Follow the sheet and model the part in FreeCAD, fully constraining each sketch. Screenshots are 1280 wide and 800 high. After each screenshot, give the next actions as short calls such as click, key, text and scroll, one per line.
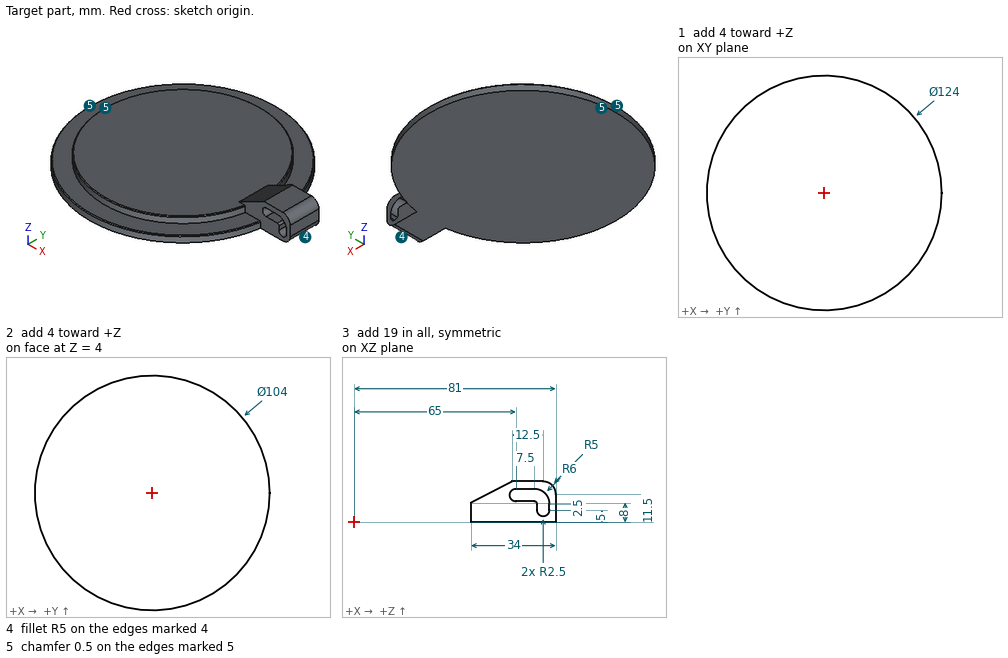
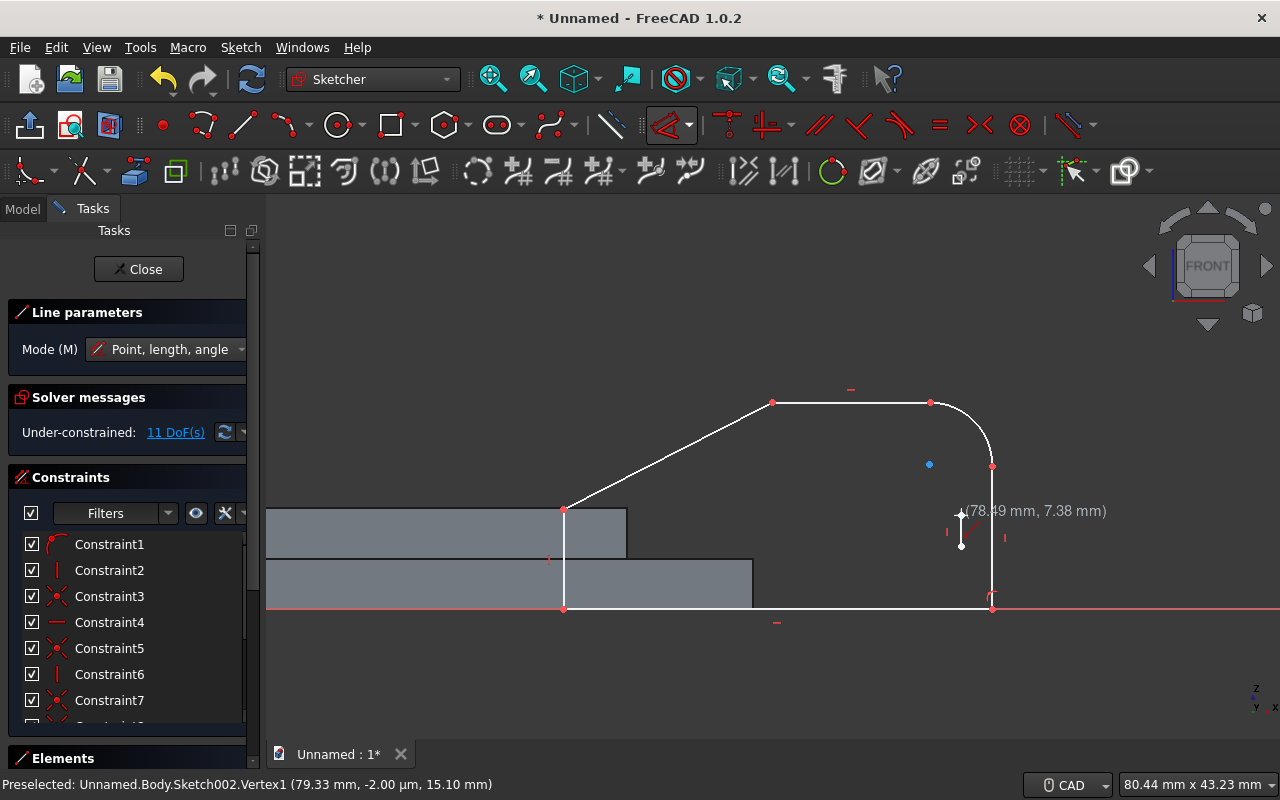
click(886, 439)
click(791, 439)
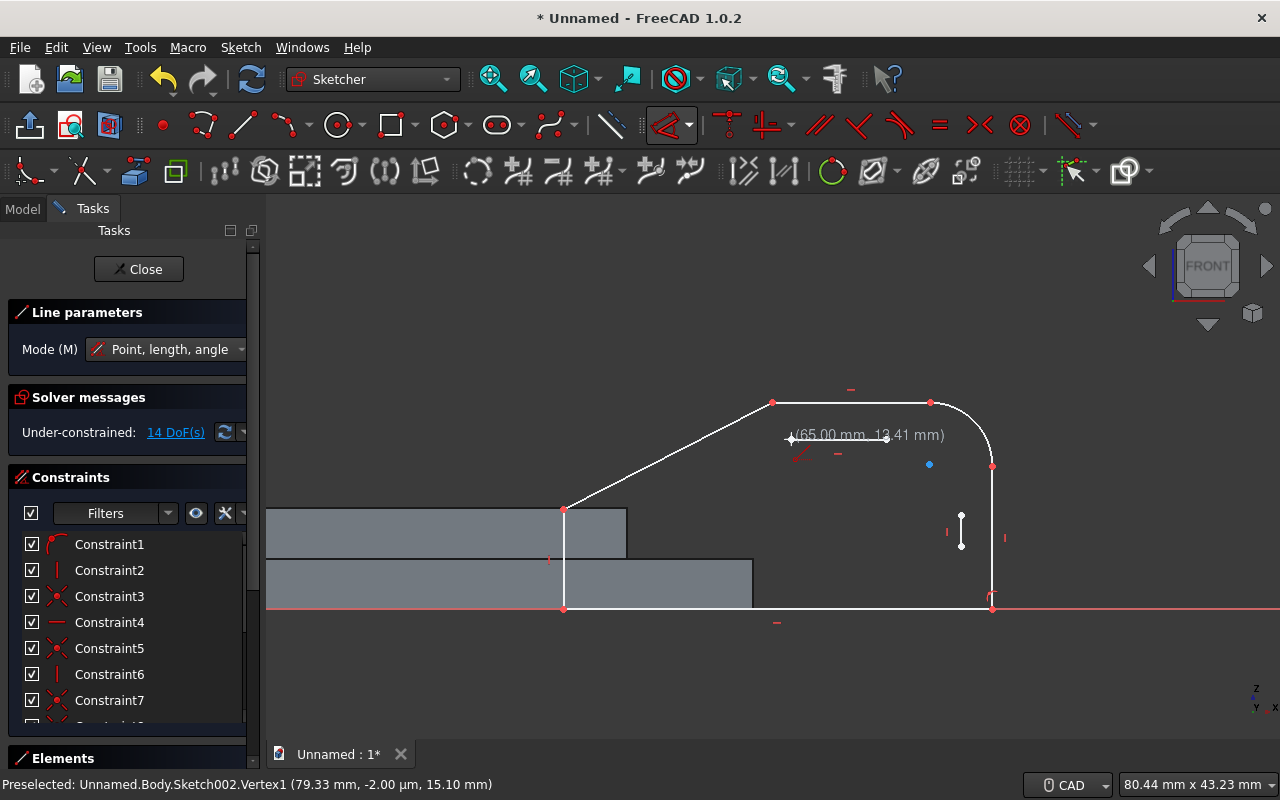
click(791, 502)
click(886, 502)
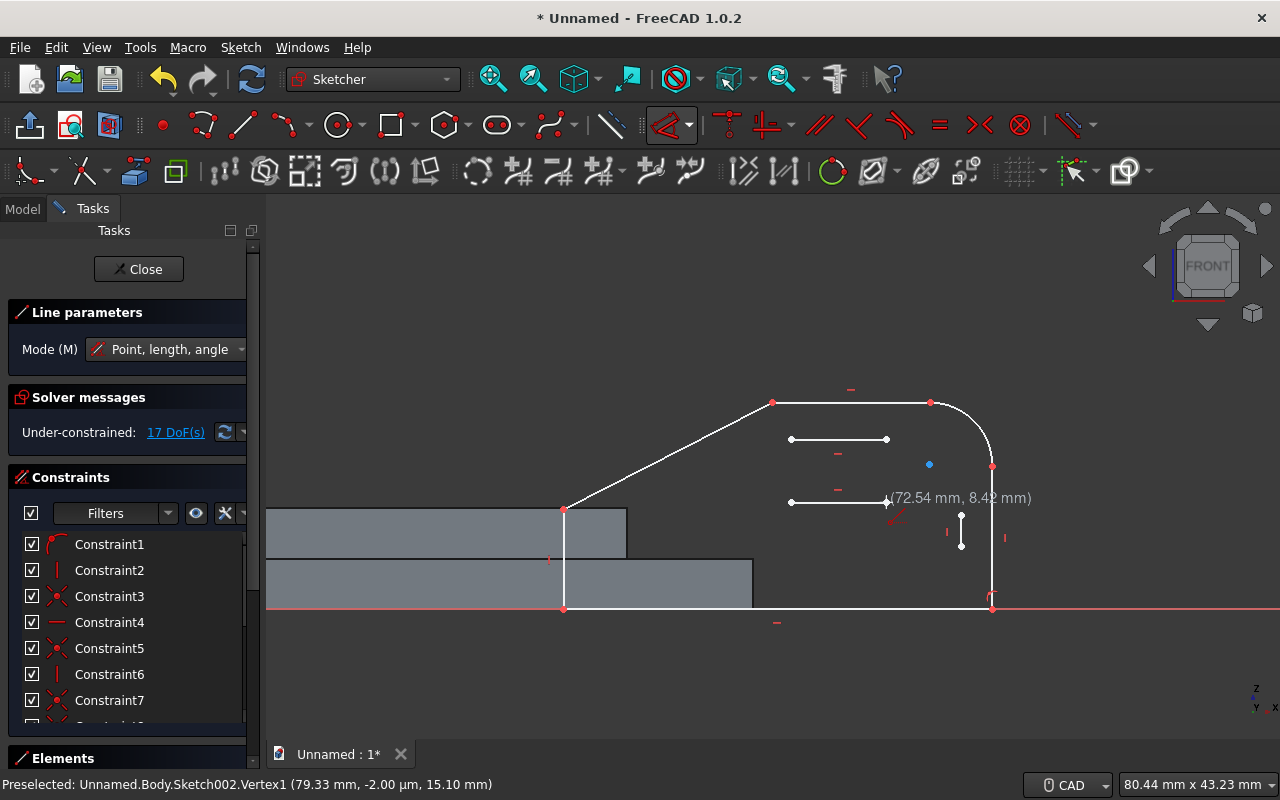
click(898, 515)
click(898, 546)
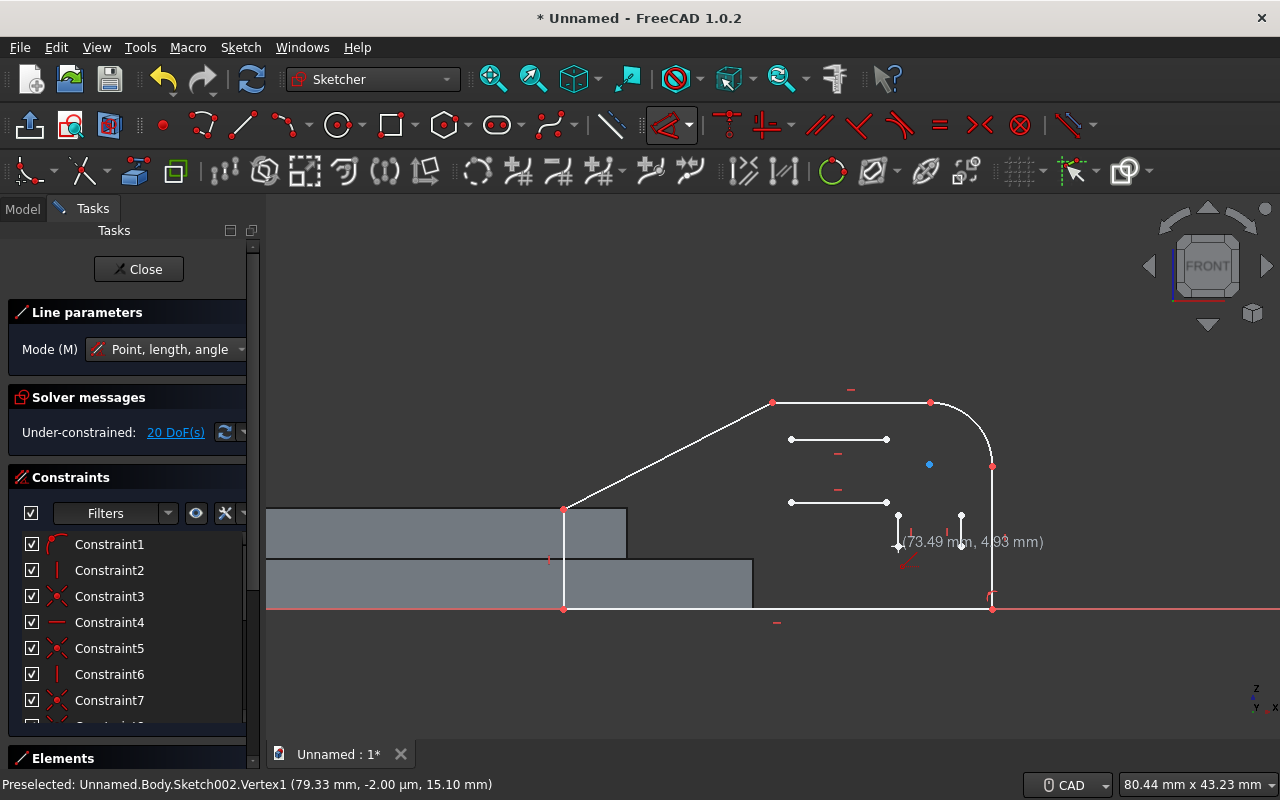
click(284, 126)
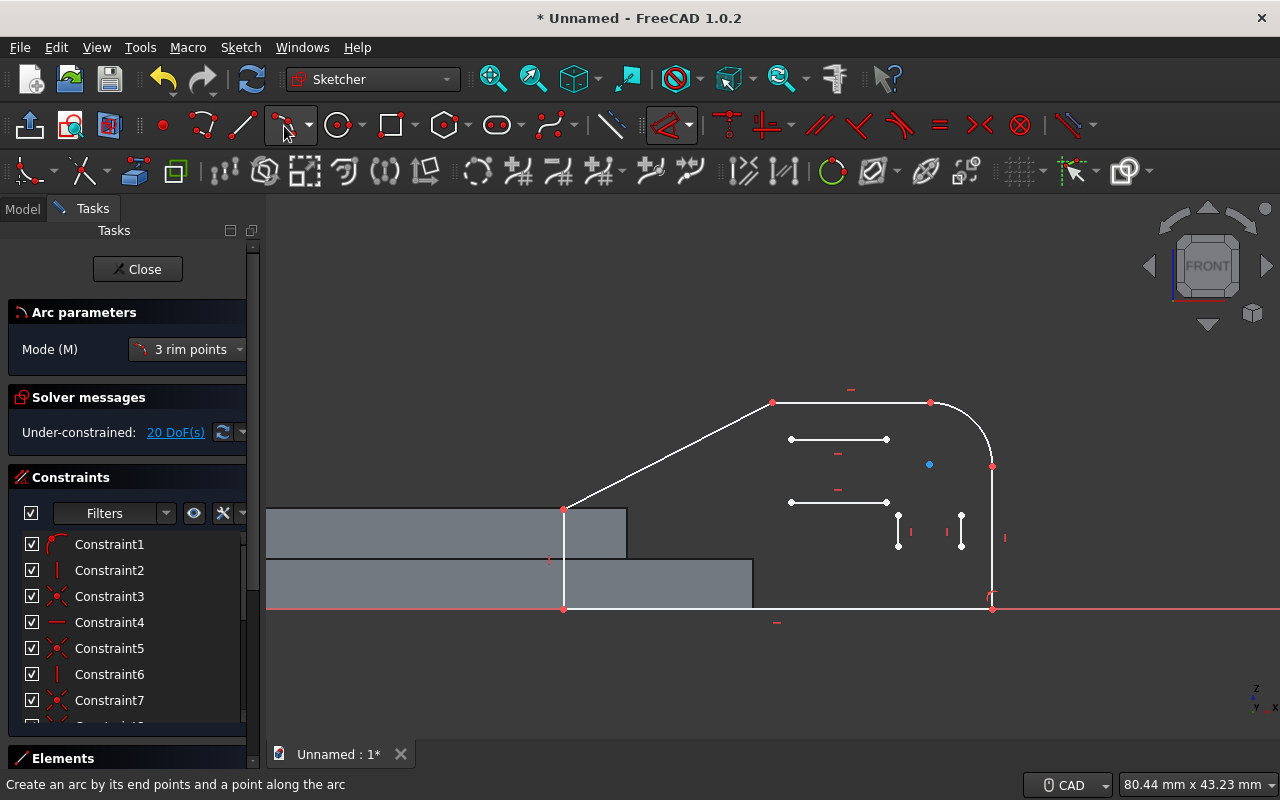
click(961, 516)
click(886, 440)
click(953, 480)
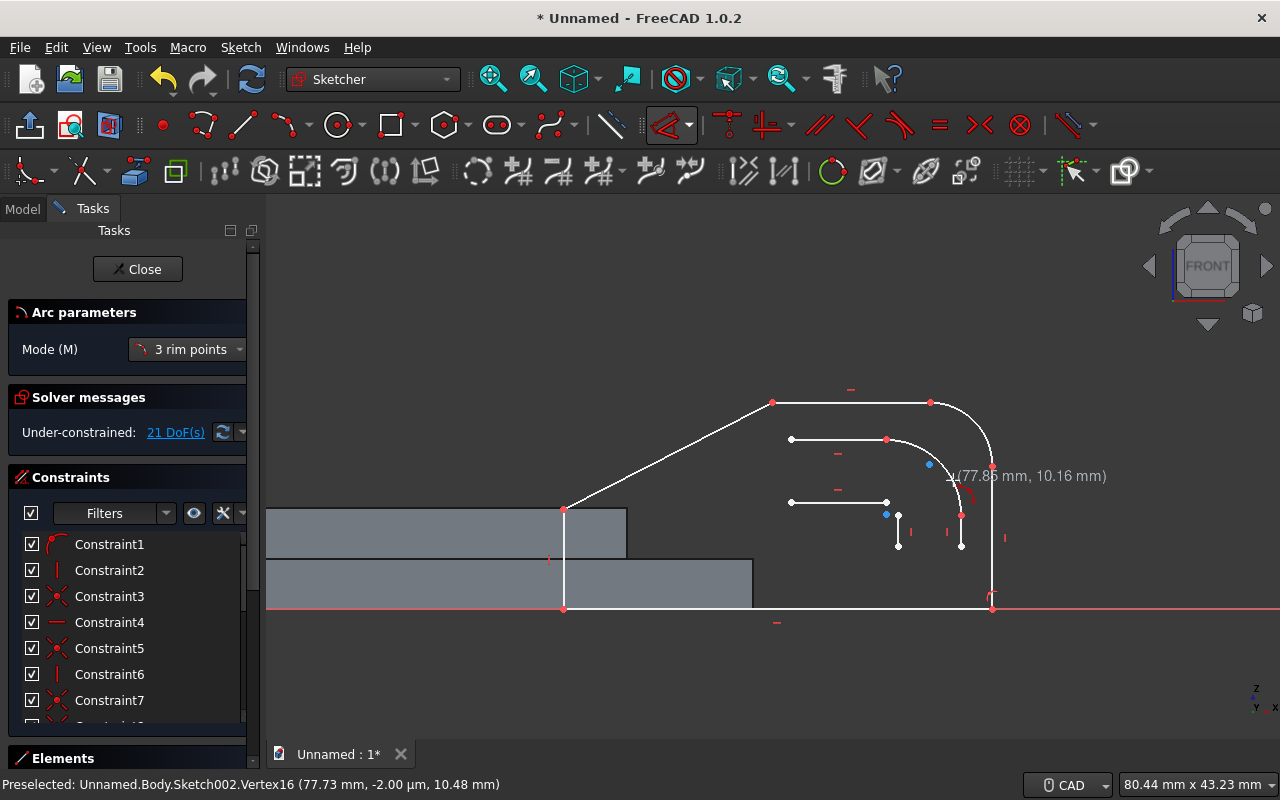
click(791, 440)
click(791, 503)
click(759, 470)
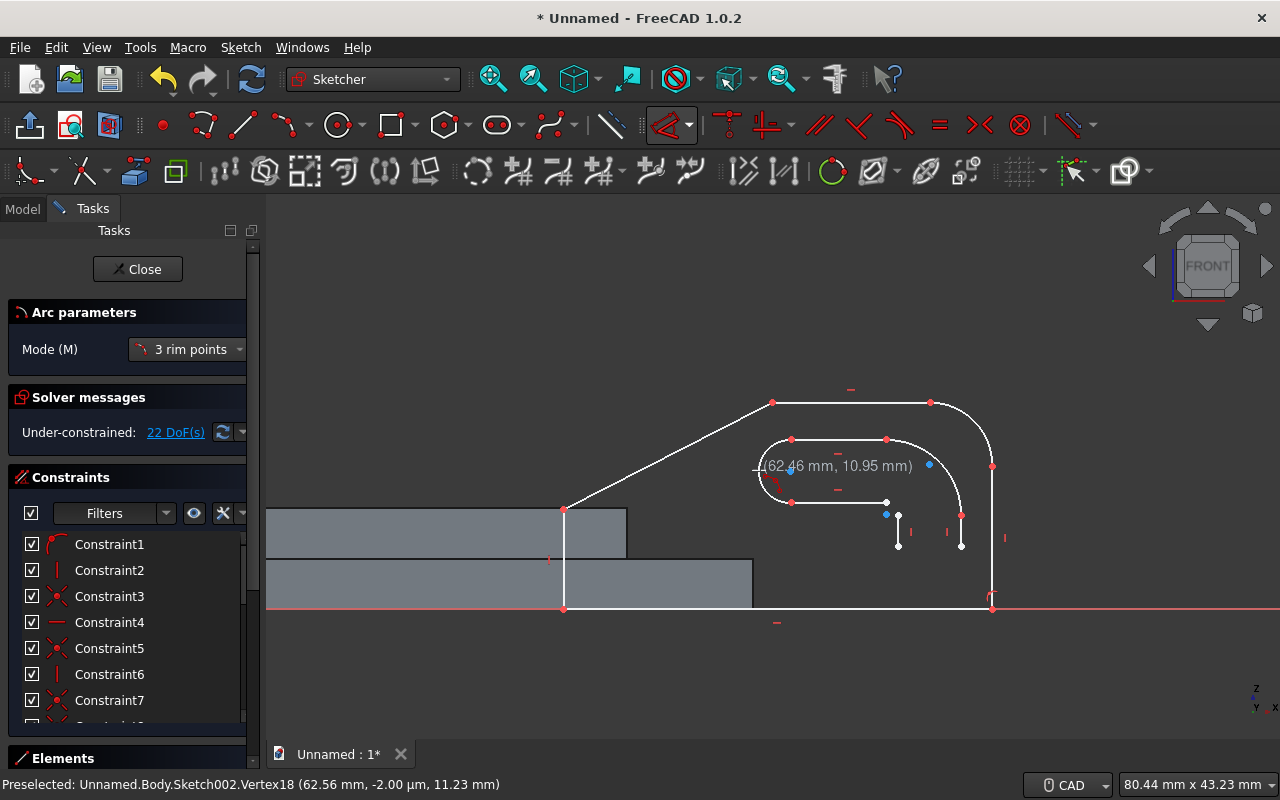
scroll(886, 502, up, 2)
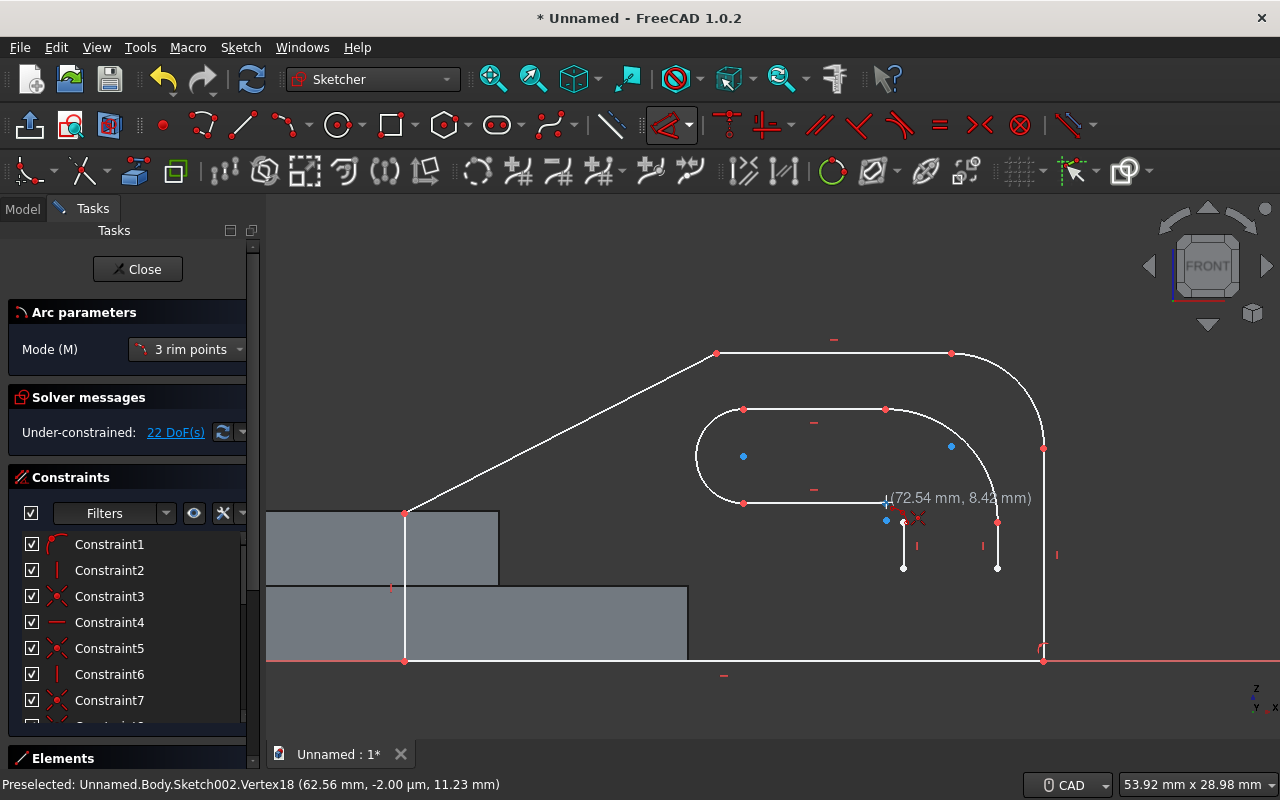
click(886, 503)
click(904, 523)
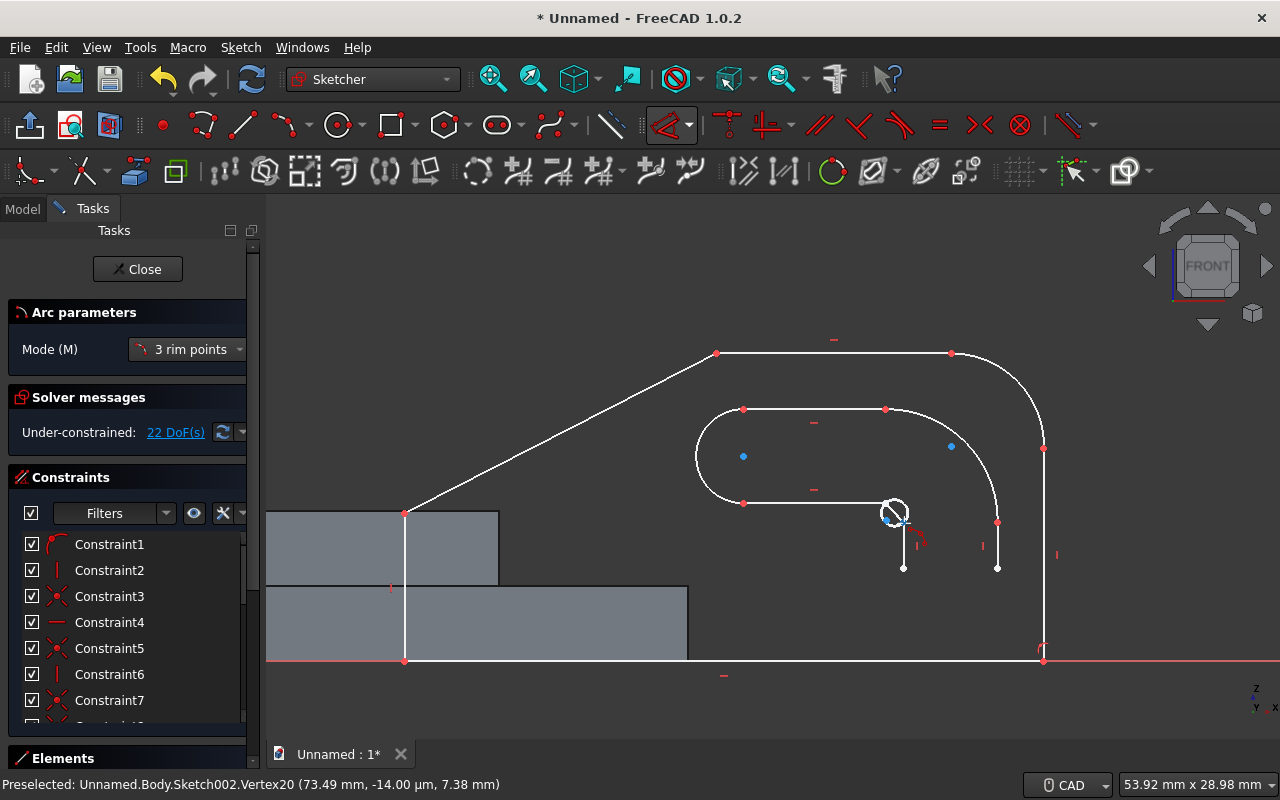
scroll(898, 507, up, 6)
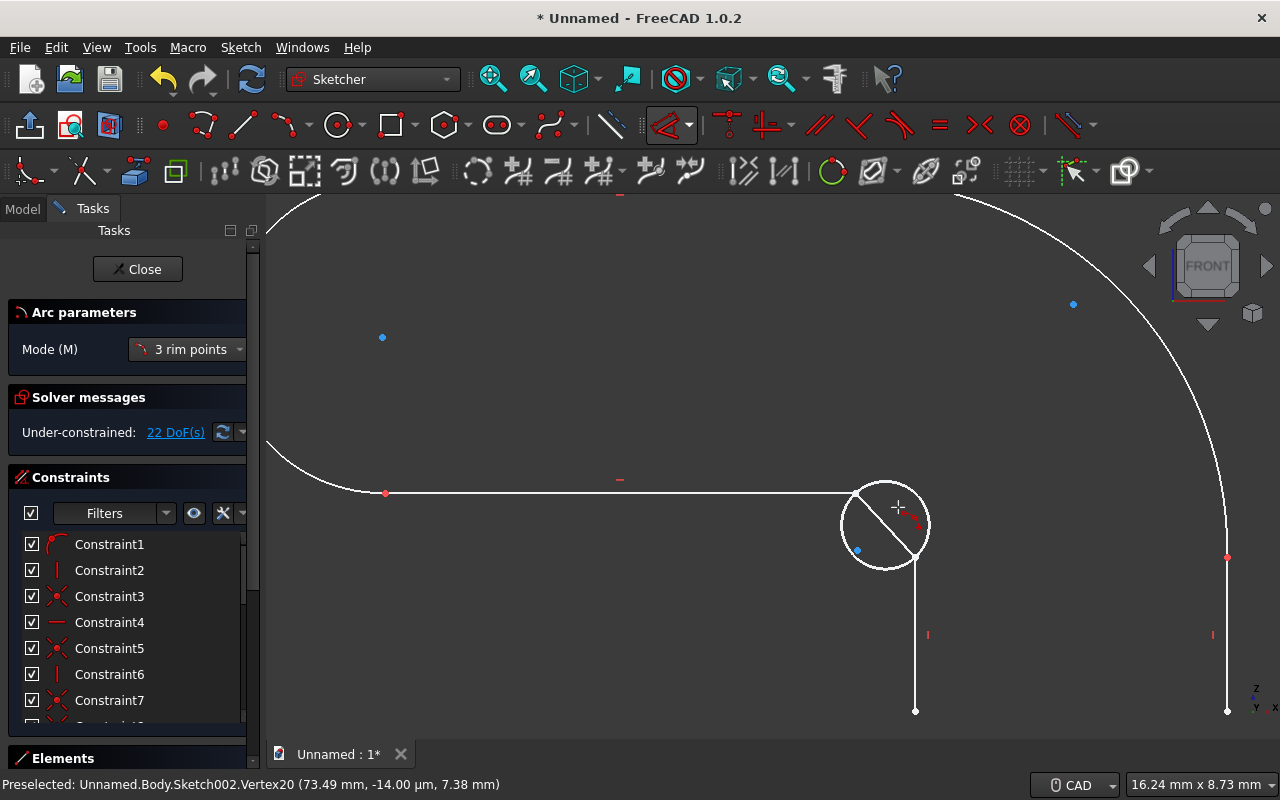
click(898, 506)